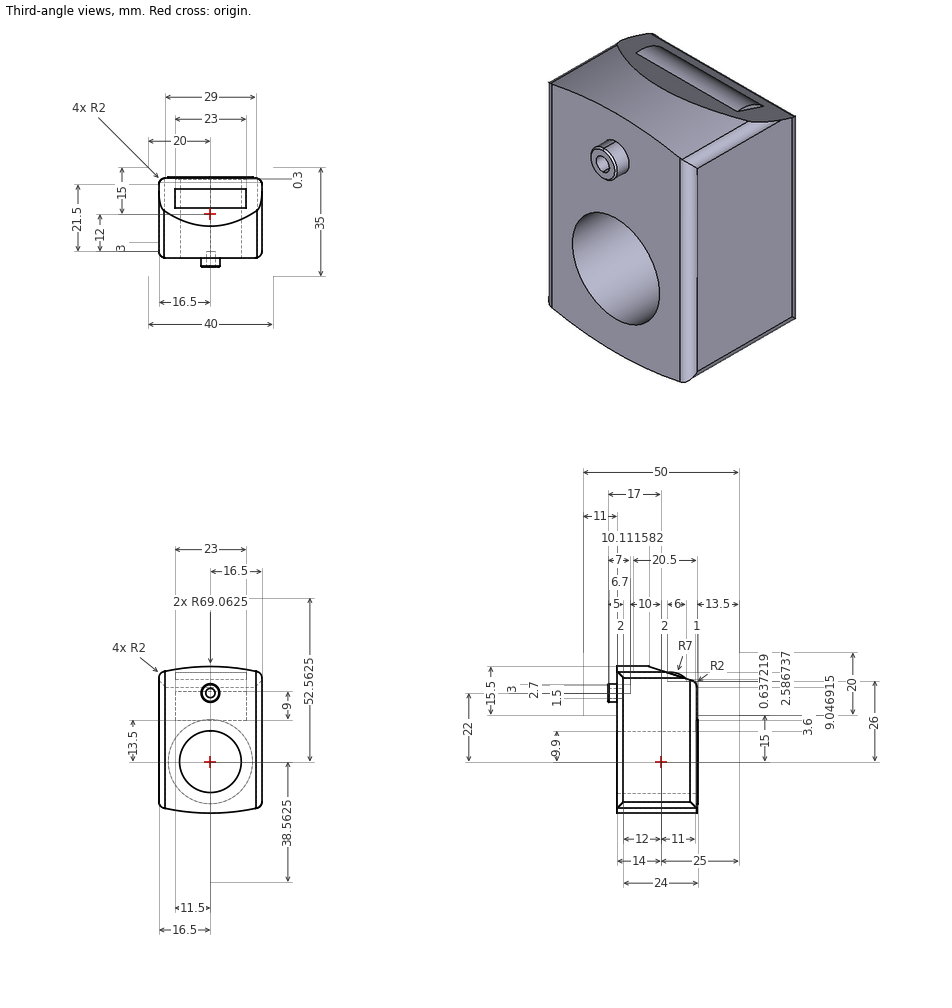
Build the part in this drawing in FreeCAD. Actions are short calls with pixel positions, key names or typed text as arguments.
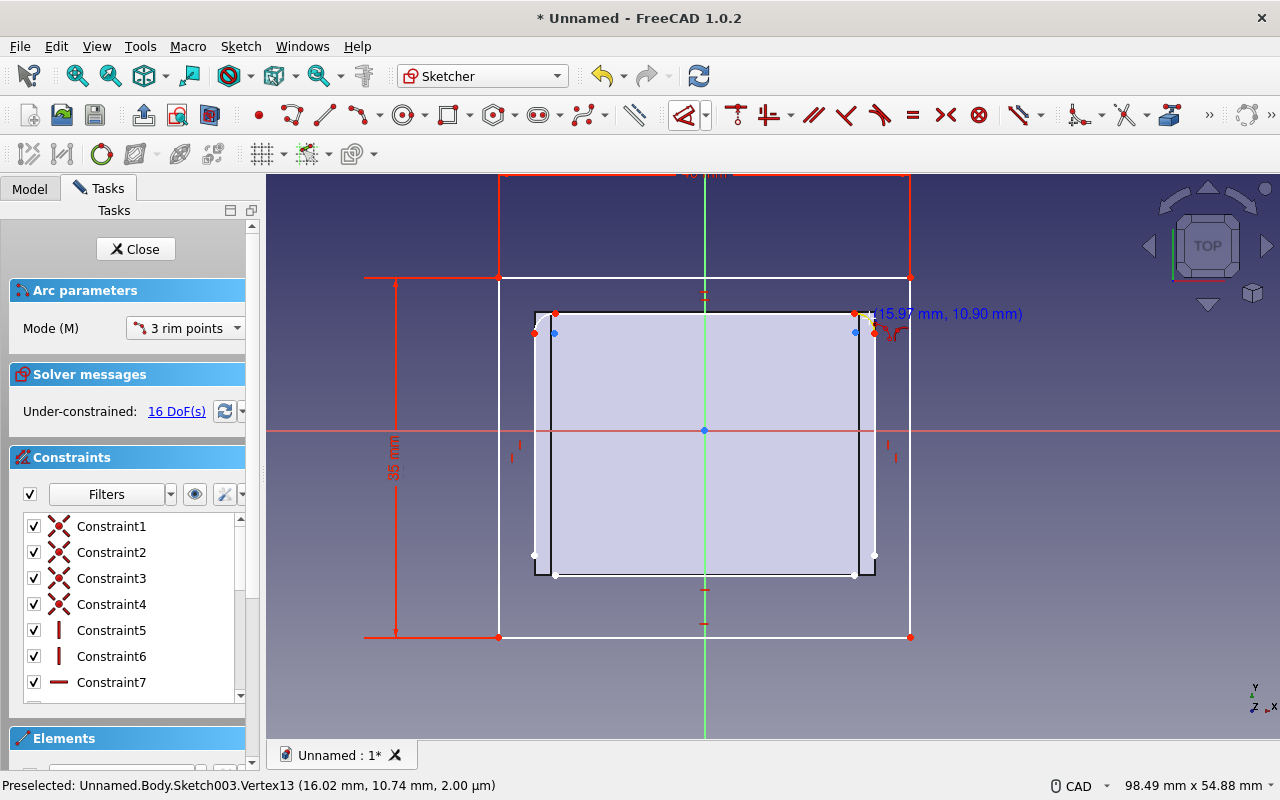
click(875, 556)
click(855, 576)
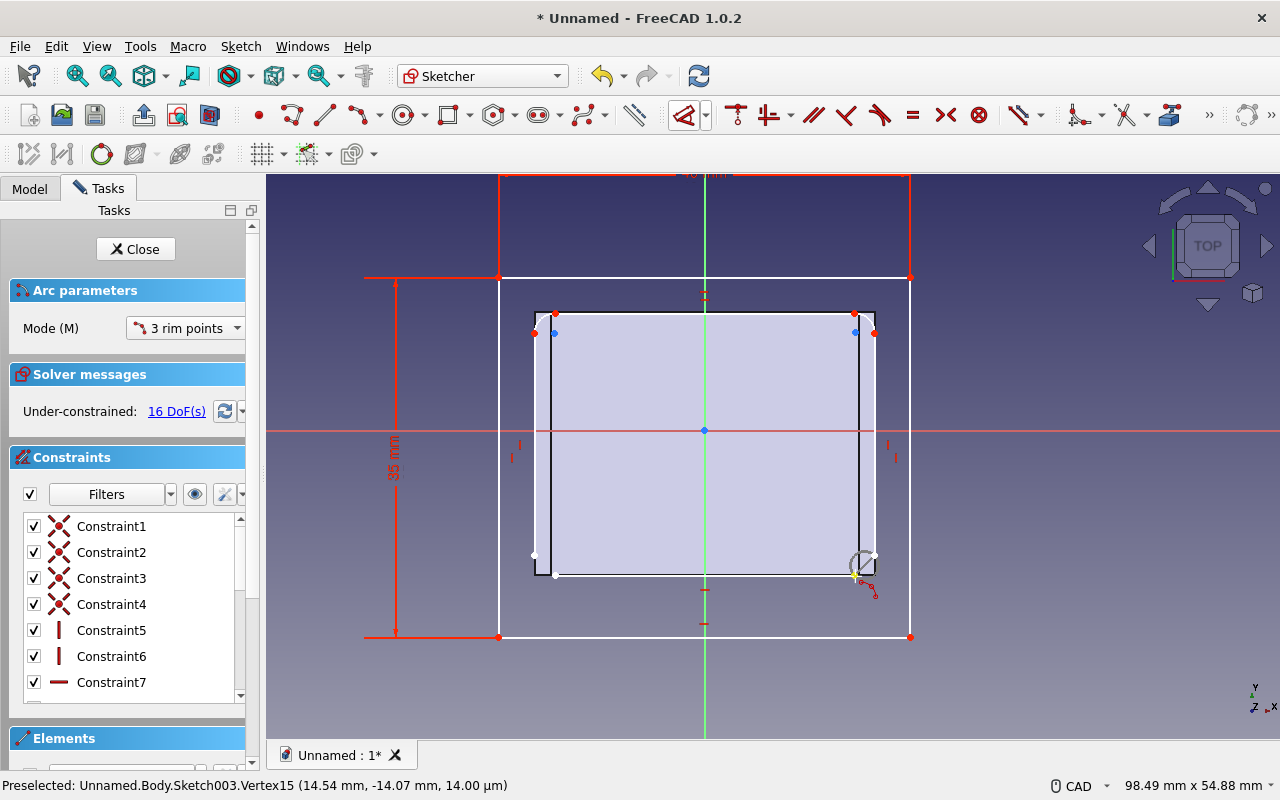
scroll(869, 569, up, 5)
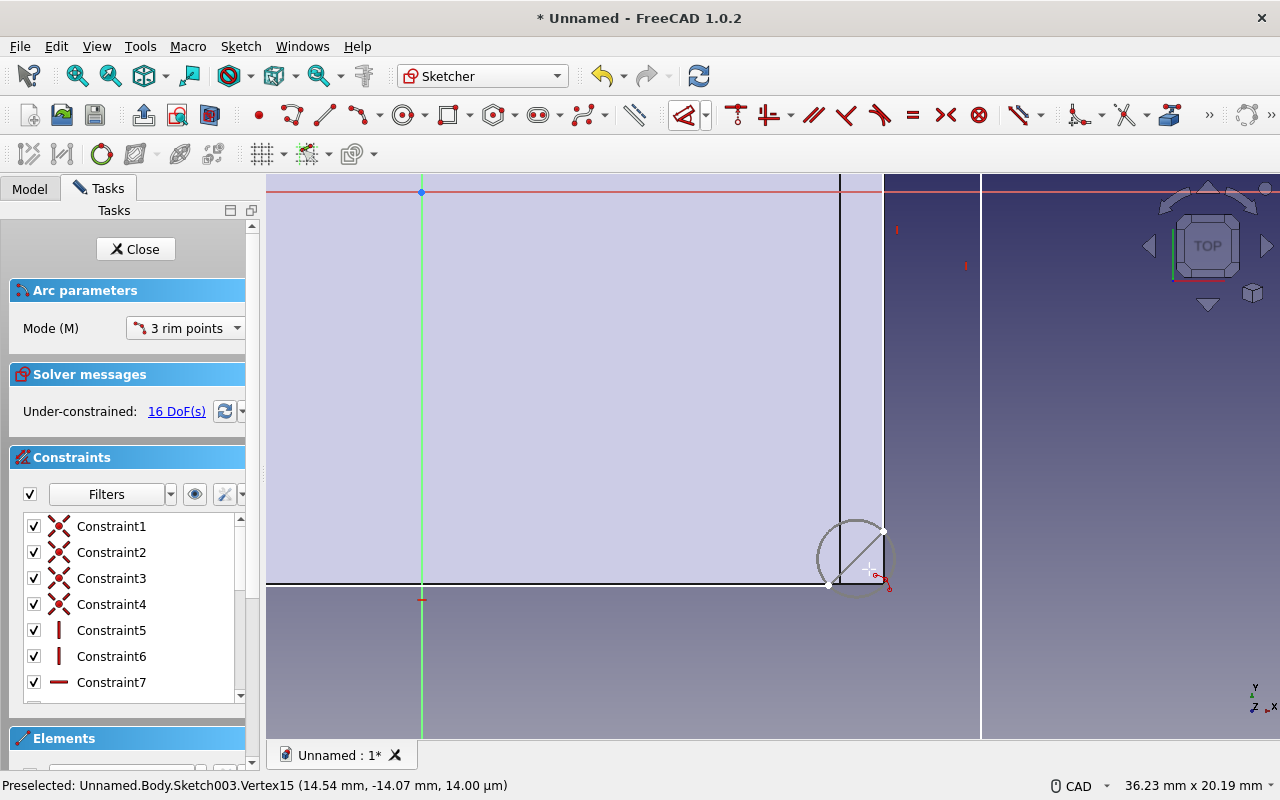
click(867, 567)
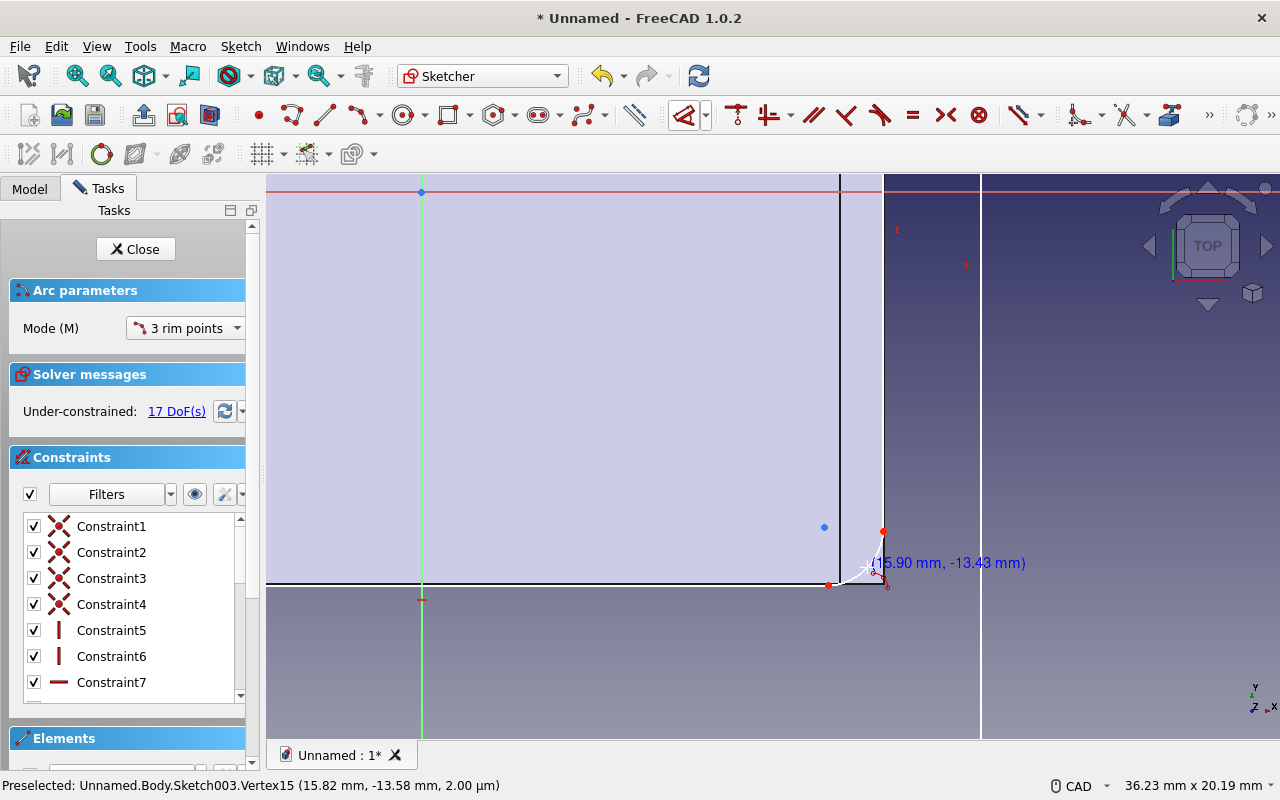
scroll(869, 570, down, 5)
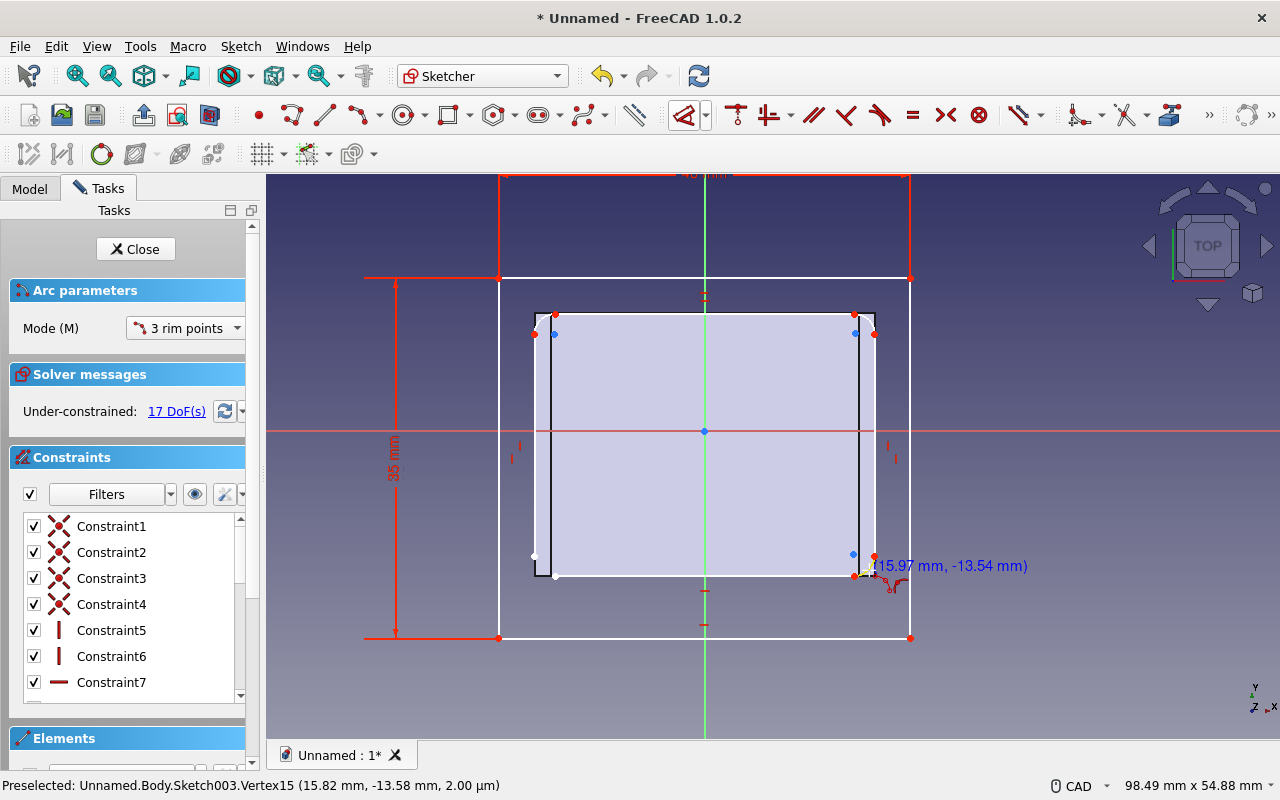
click(556, 576)
click(535, 556)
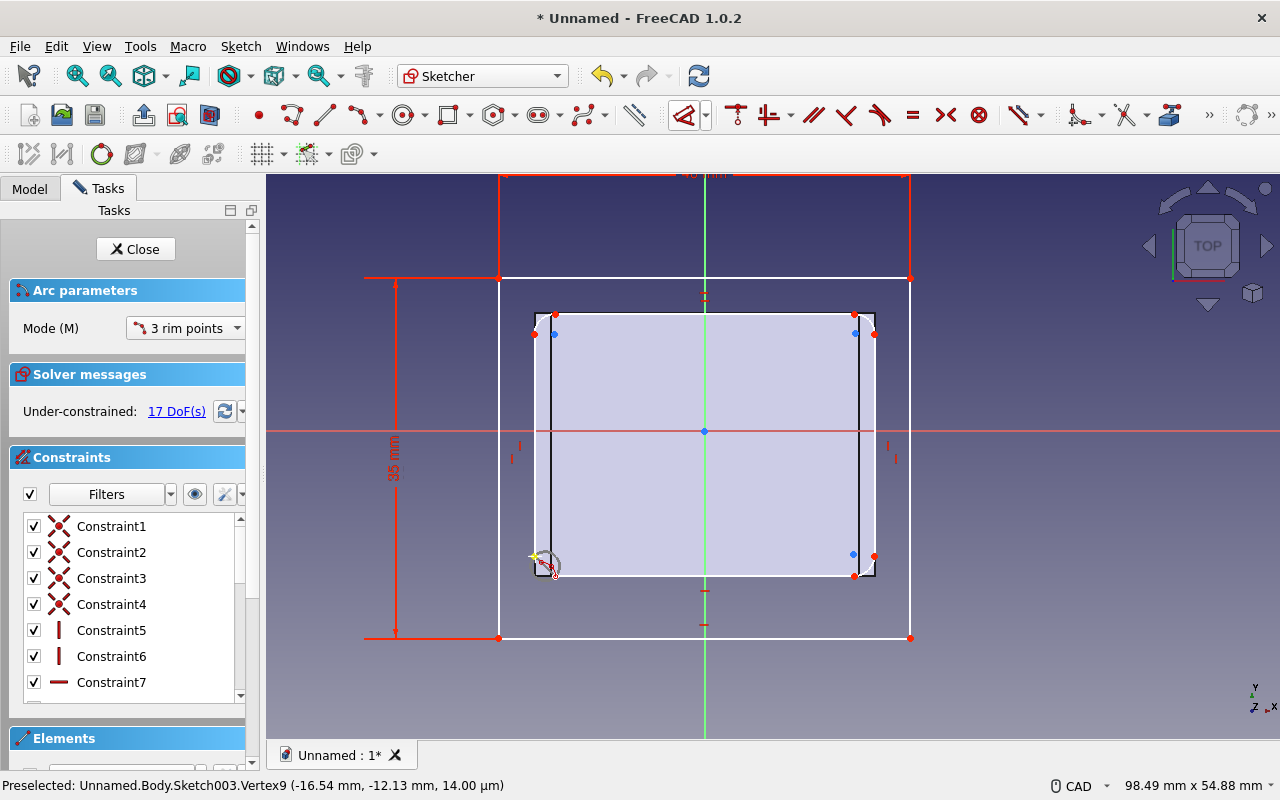
scroll(541, 570, up, 5)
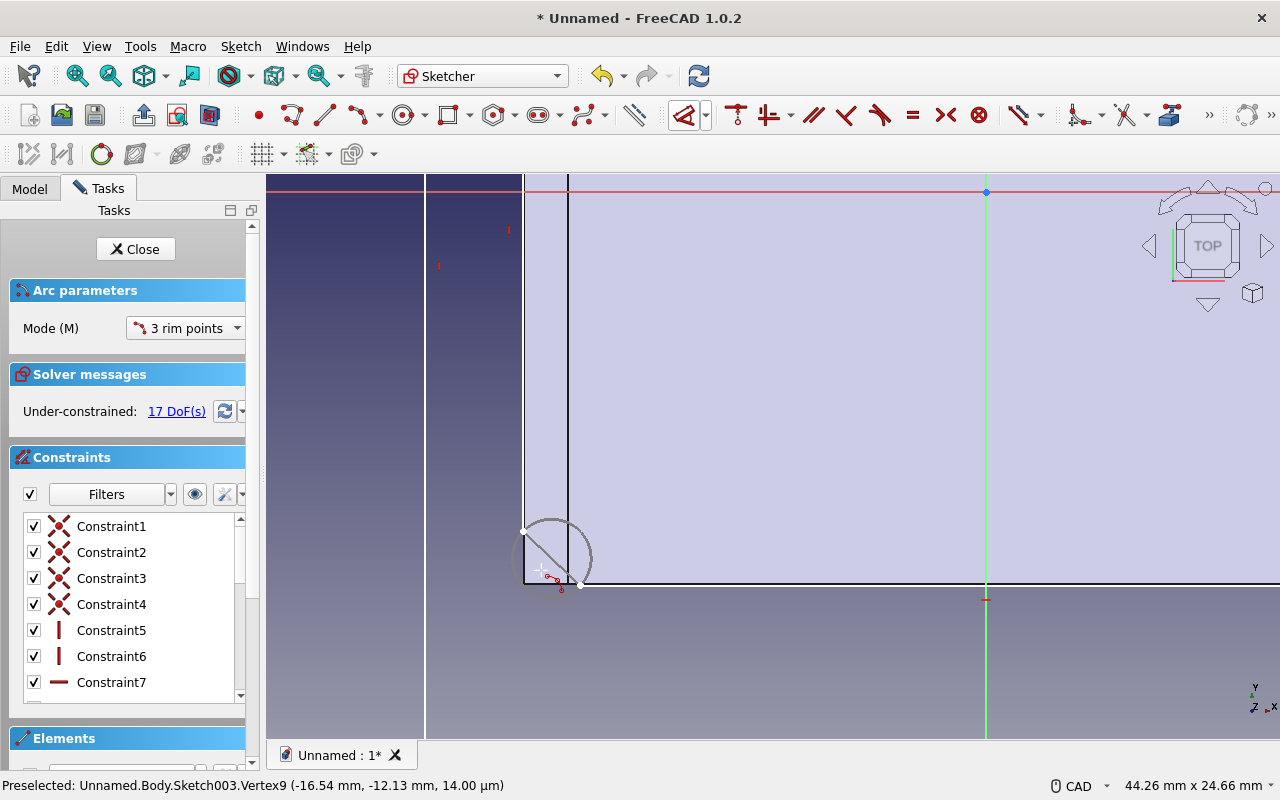
click(541, 567)
key(Escape)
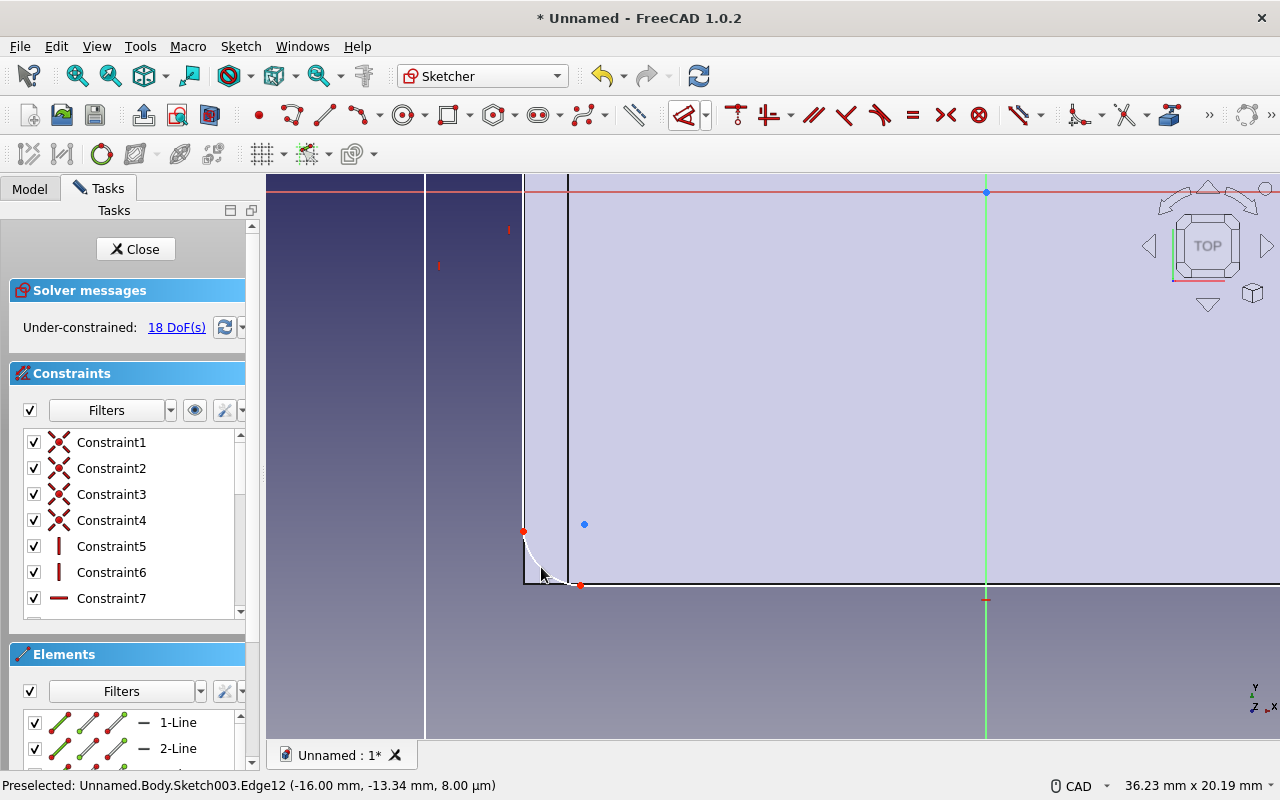
click(523, 350)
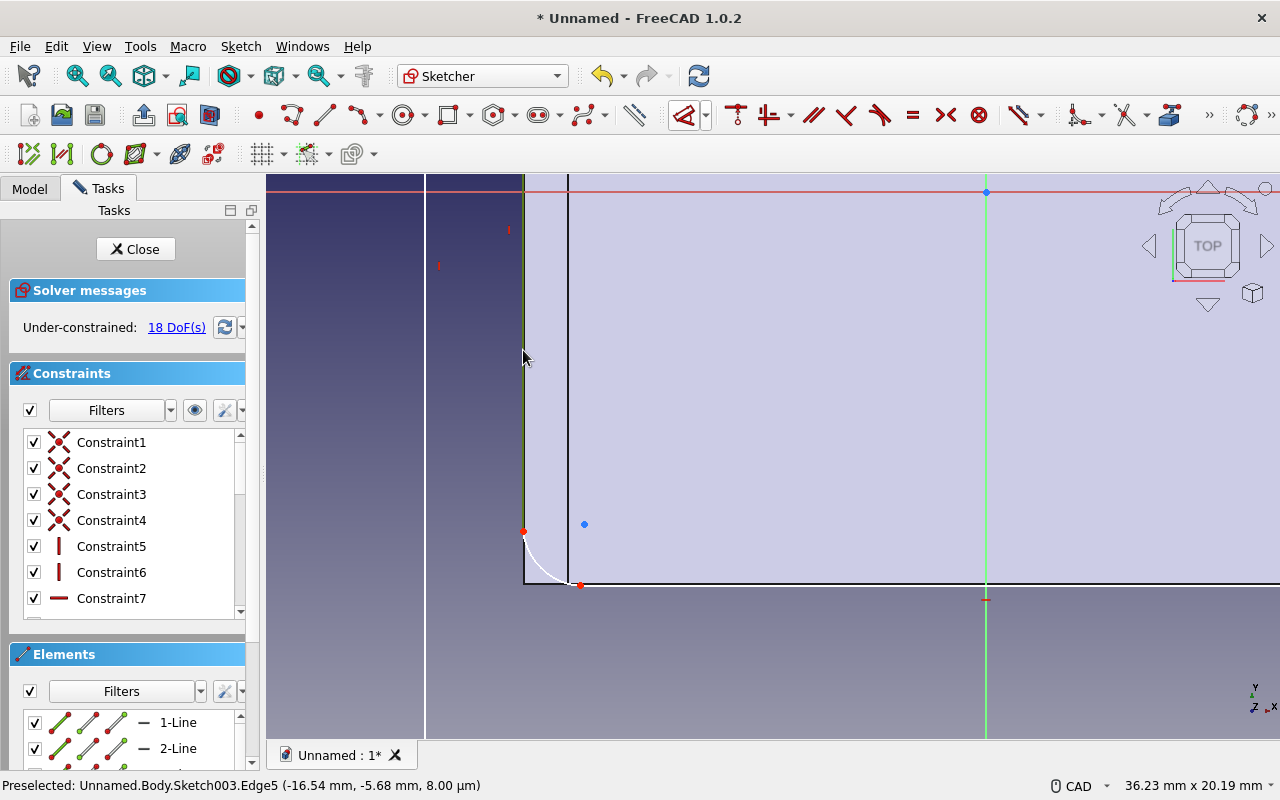
scroll(541, 570, down, 5)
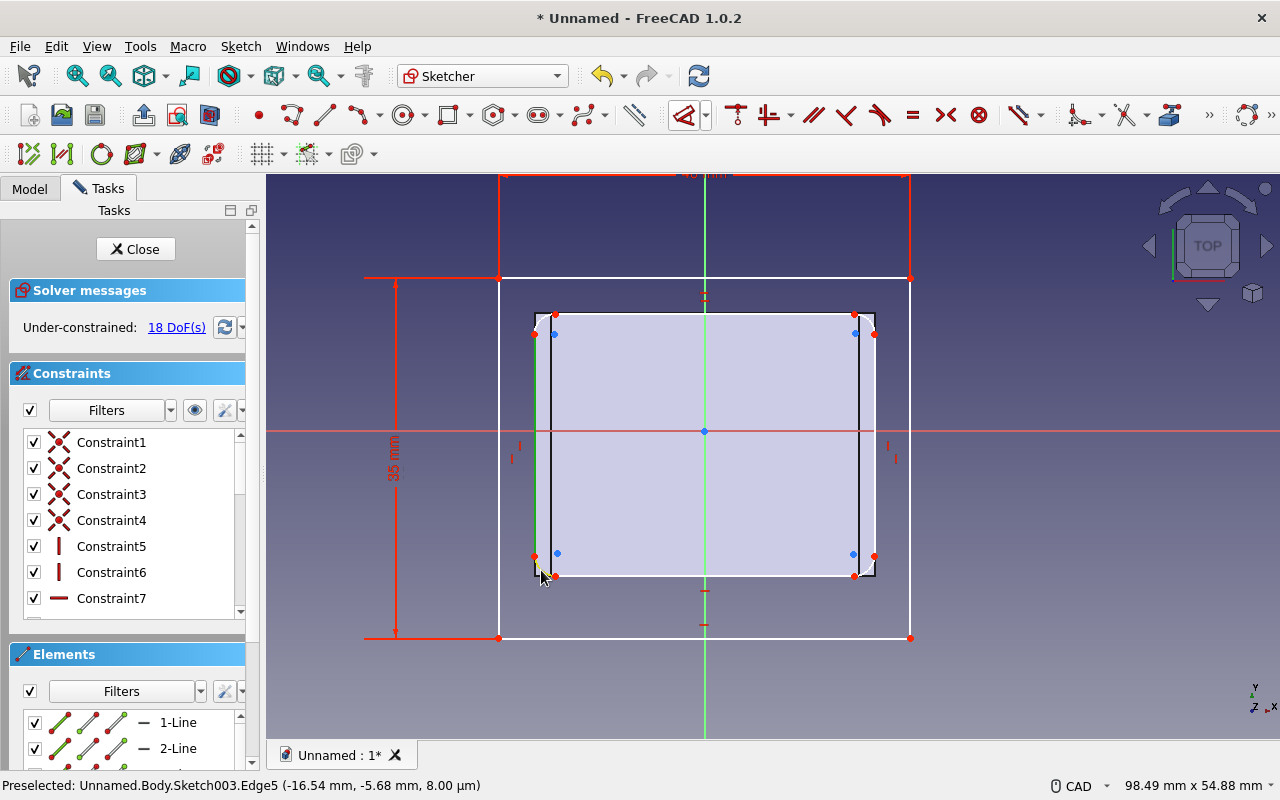
scroll(546, 316, up, 2)